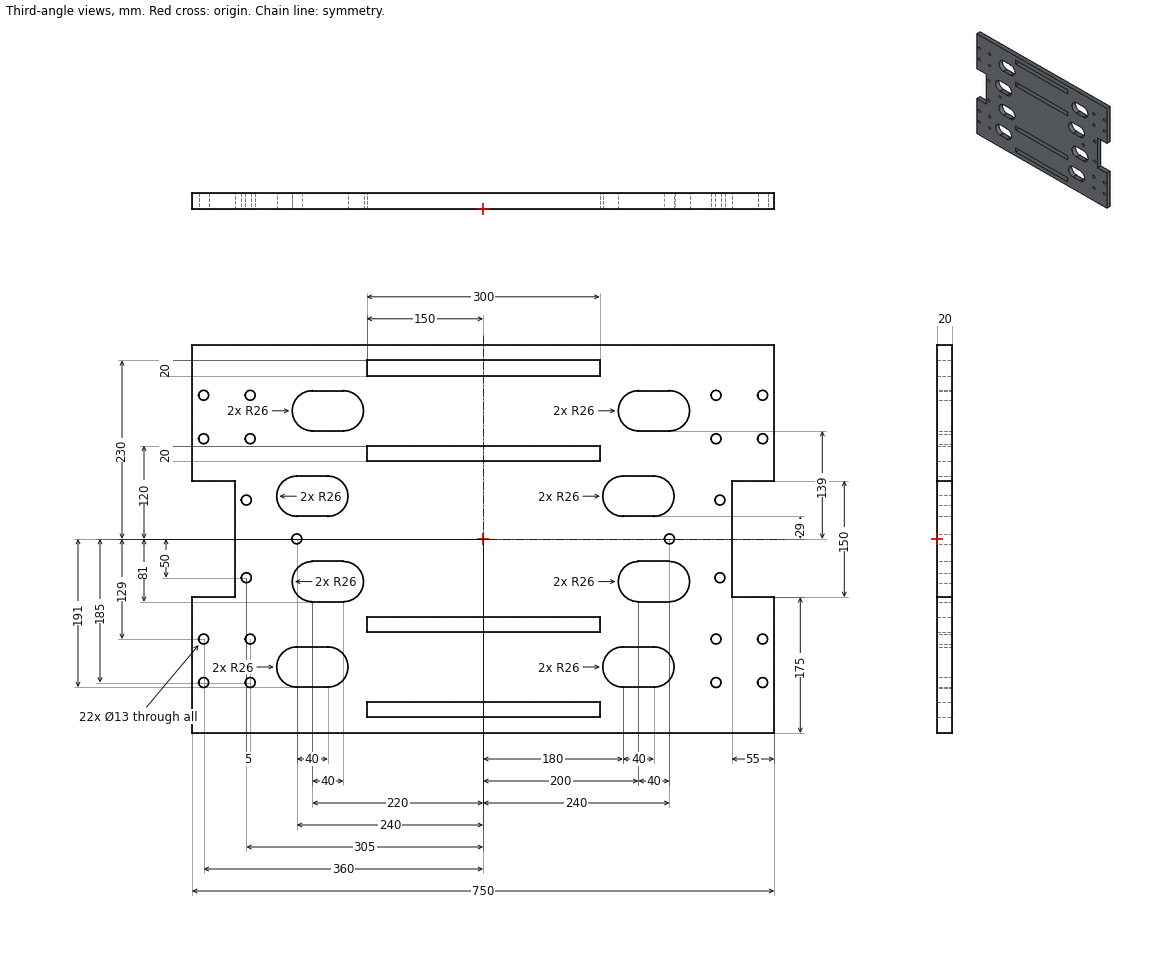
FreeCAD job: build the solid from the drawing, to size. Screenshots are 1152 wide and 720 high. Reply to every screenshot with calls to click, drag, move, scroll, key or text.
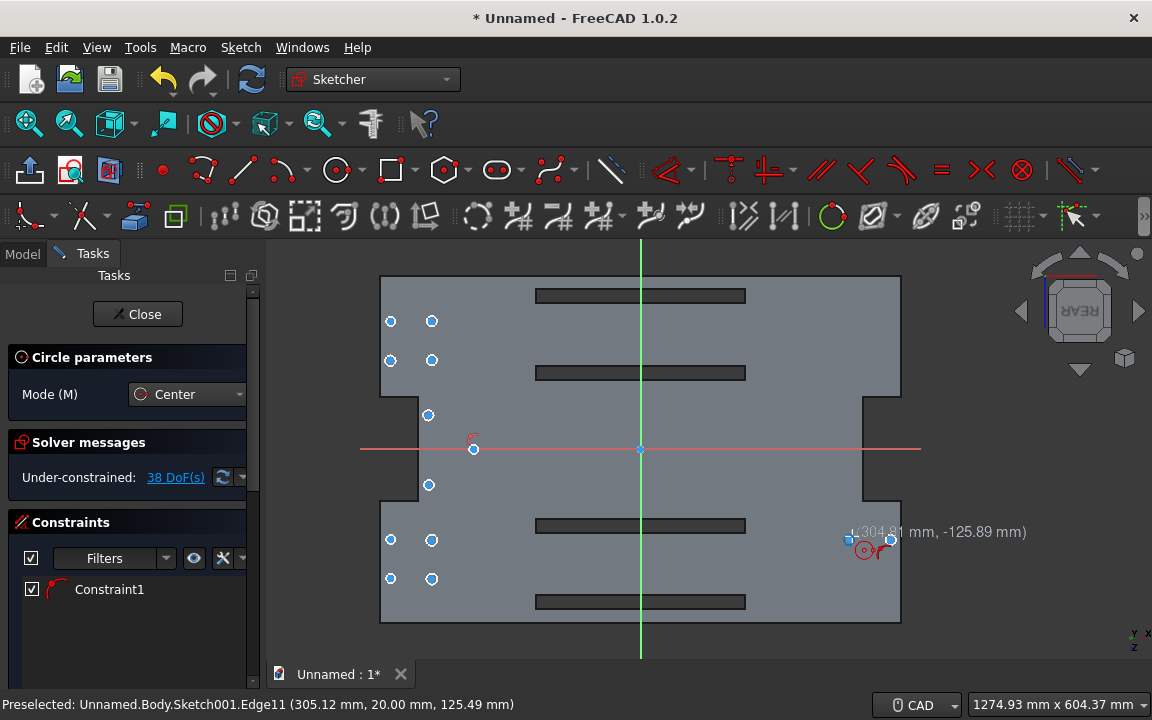
scroll(891, 578, up, 9)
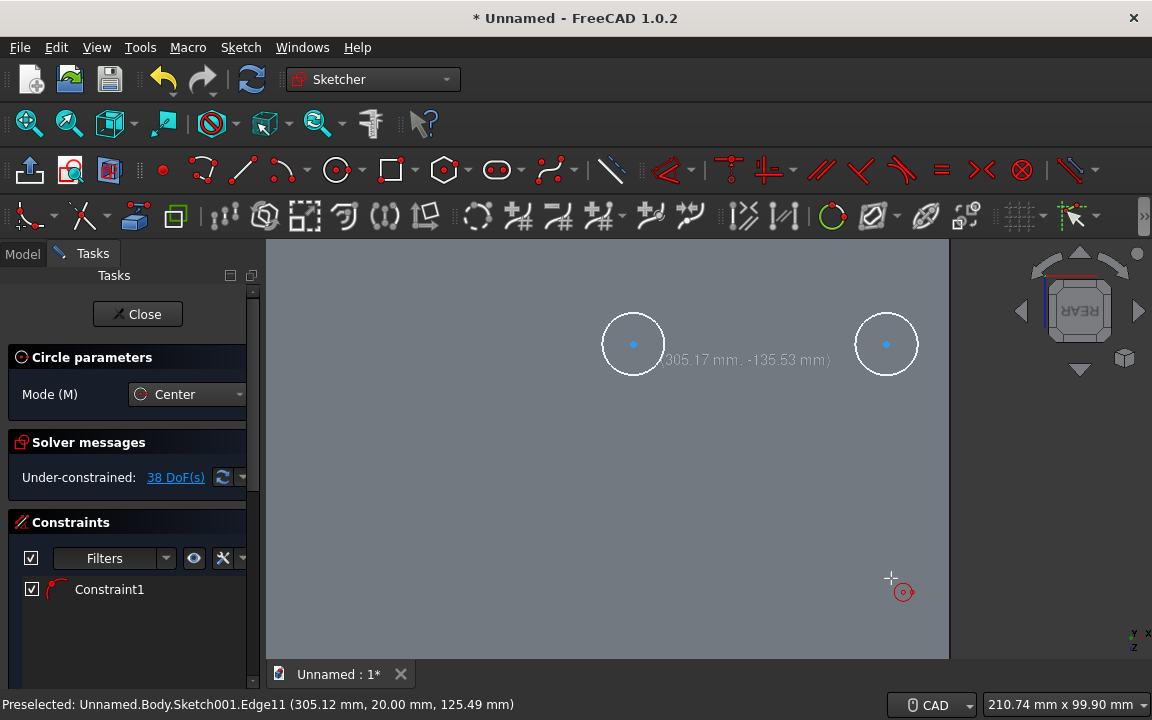
scroll(891, 578, down, 9)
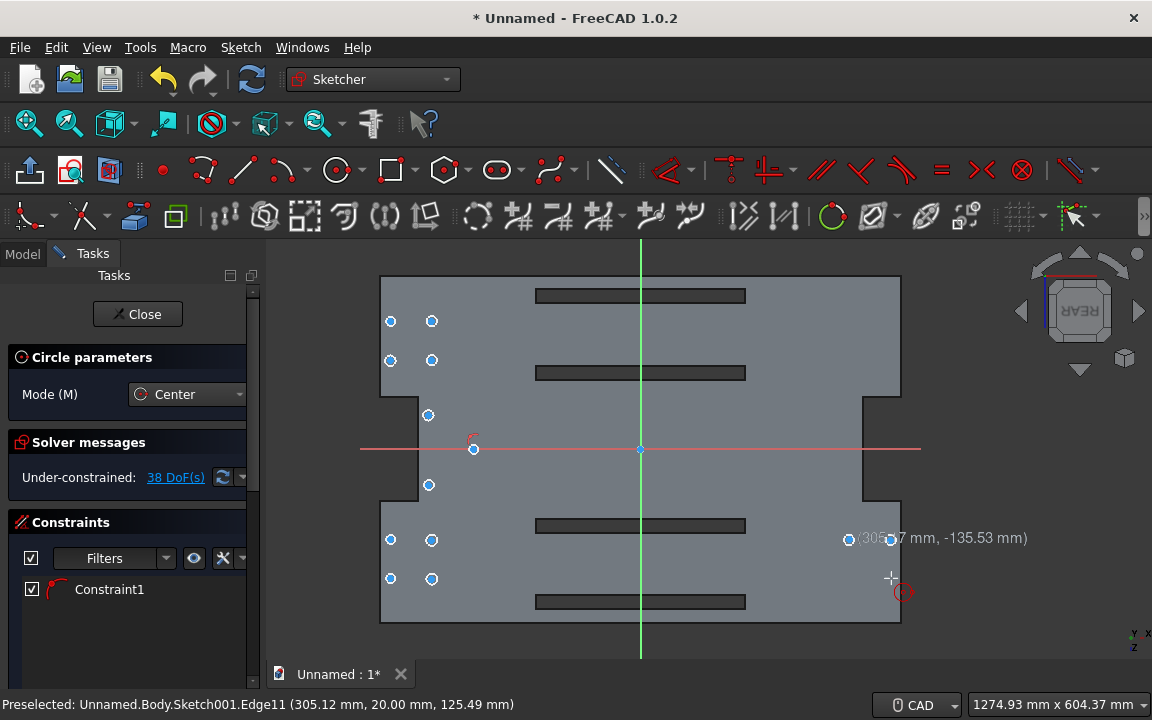
click(891, 578)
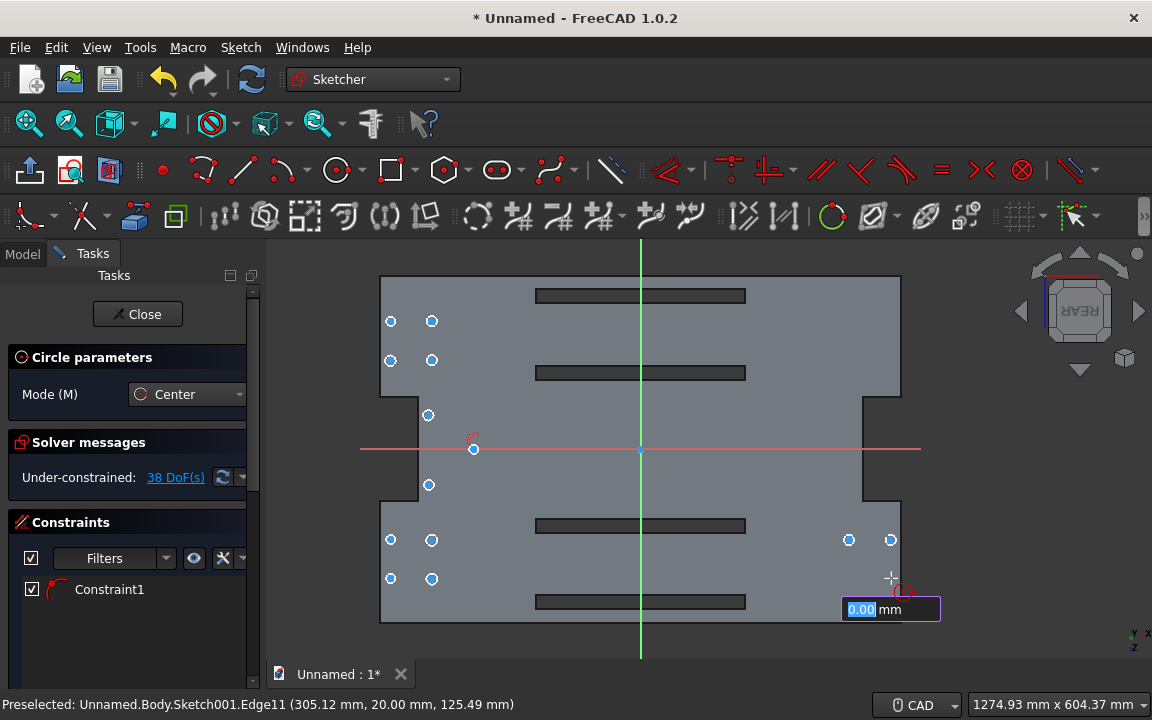
scroll(894, 575, up, 7)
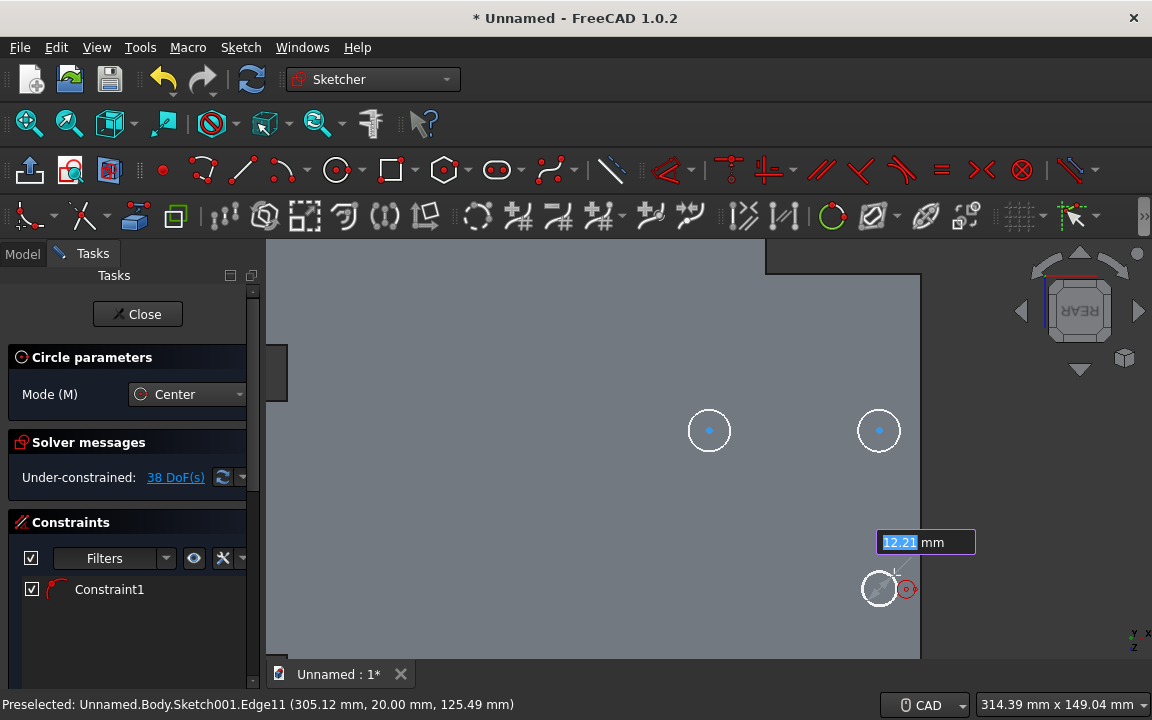
click(892, 571)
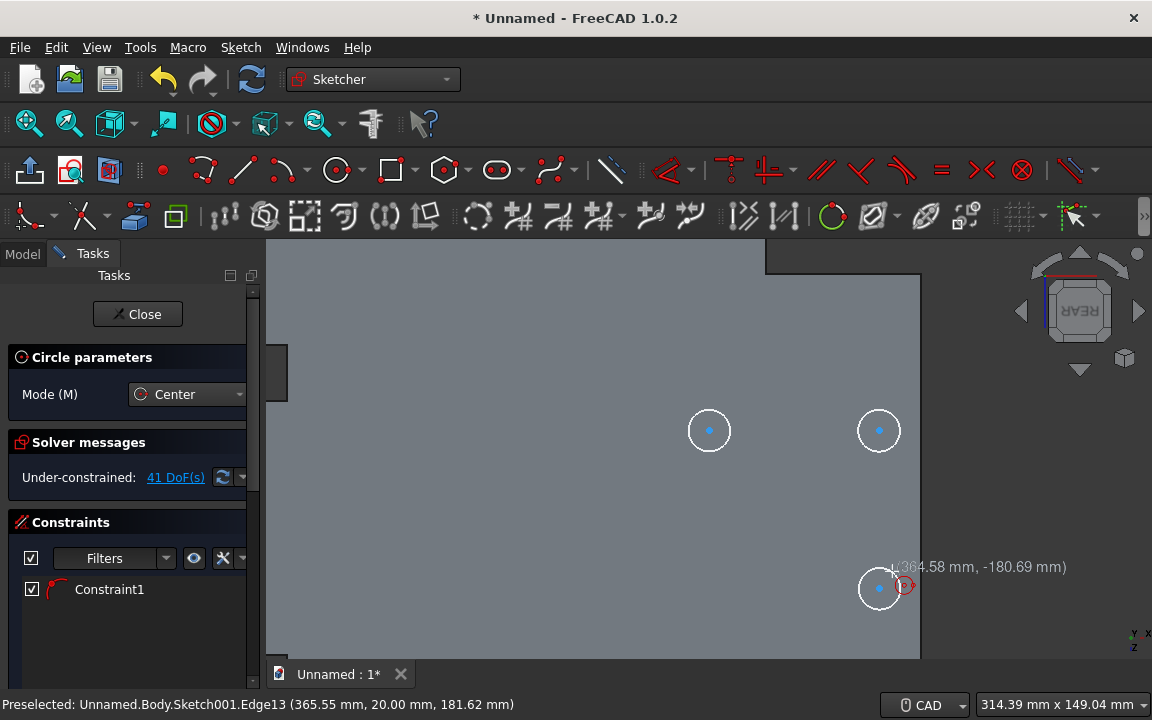
scroll(894, 575, down, 7)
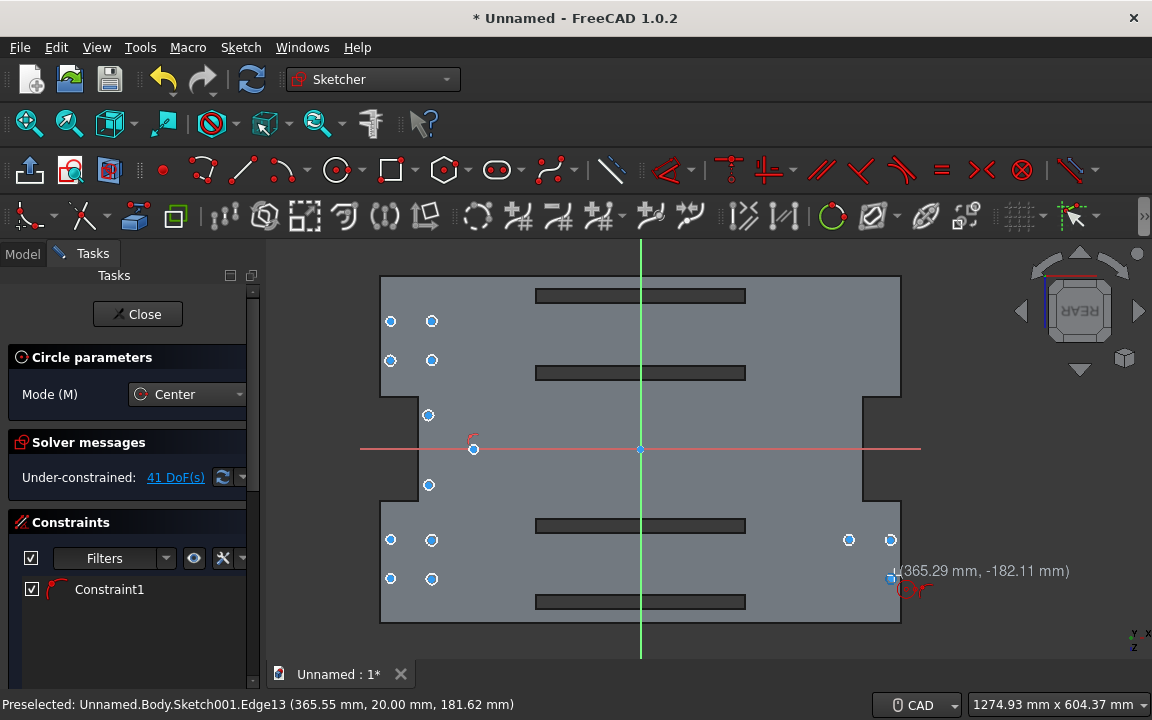
scroll(891, 360, up, 9)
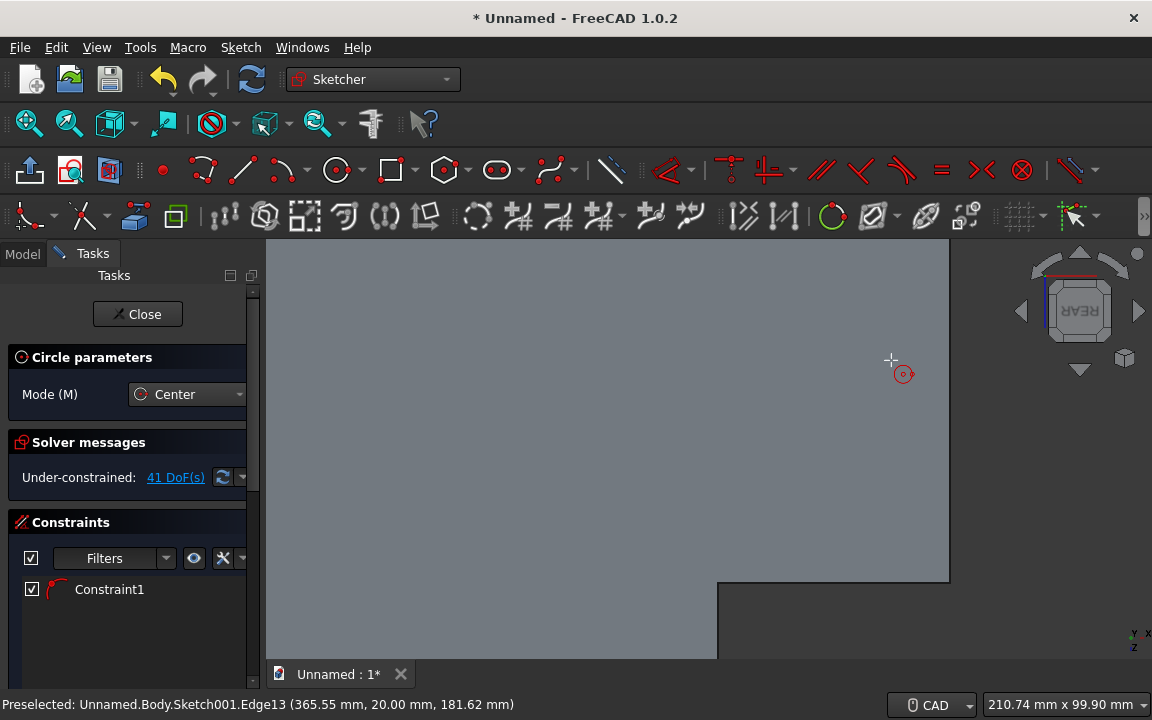
scroll(891, 360, down, 9)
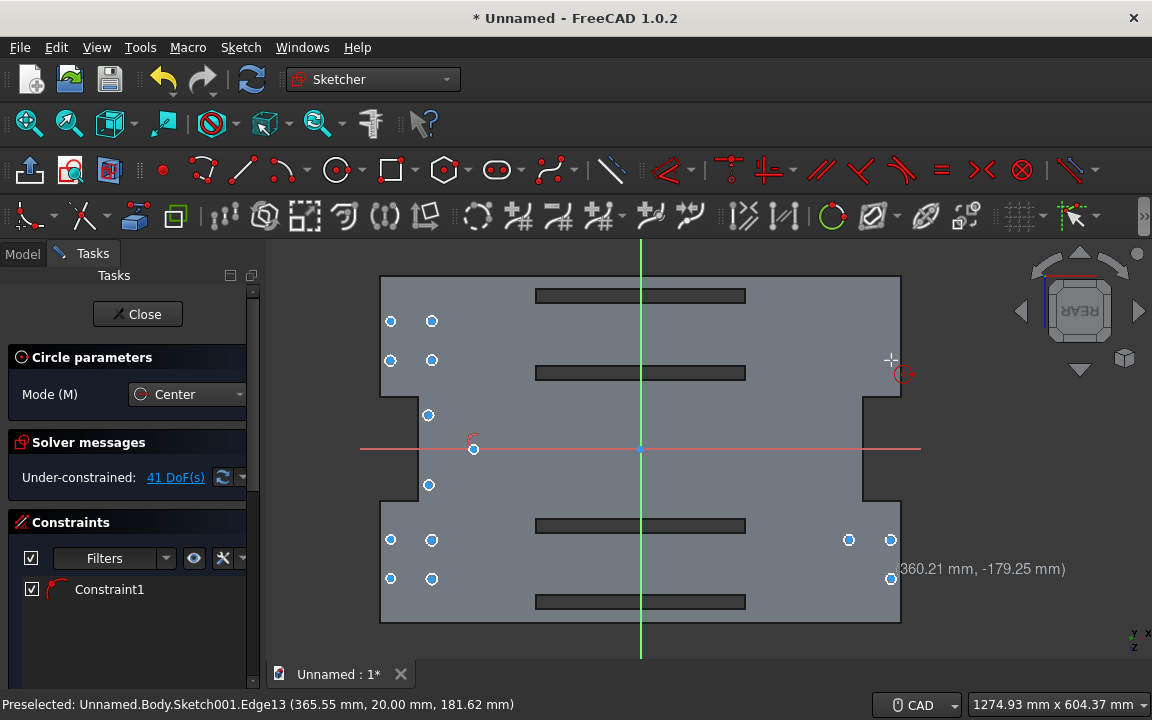
click(891, 360)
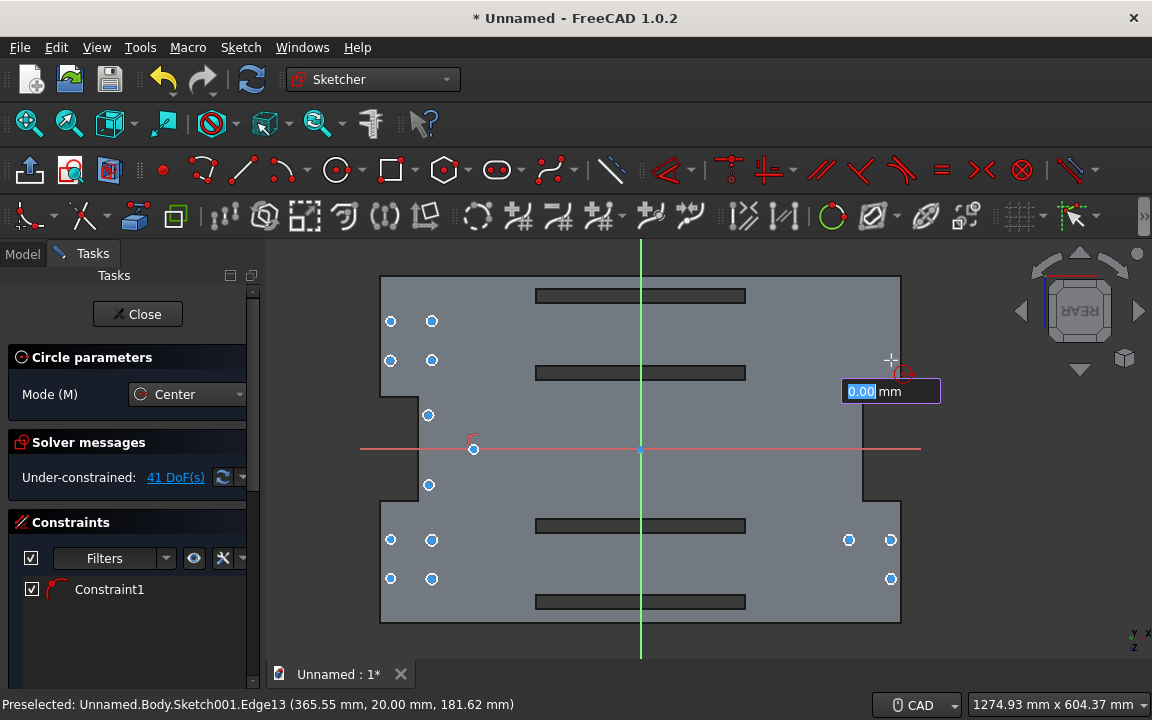
scroll(894, 356, up, 7)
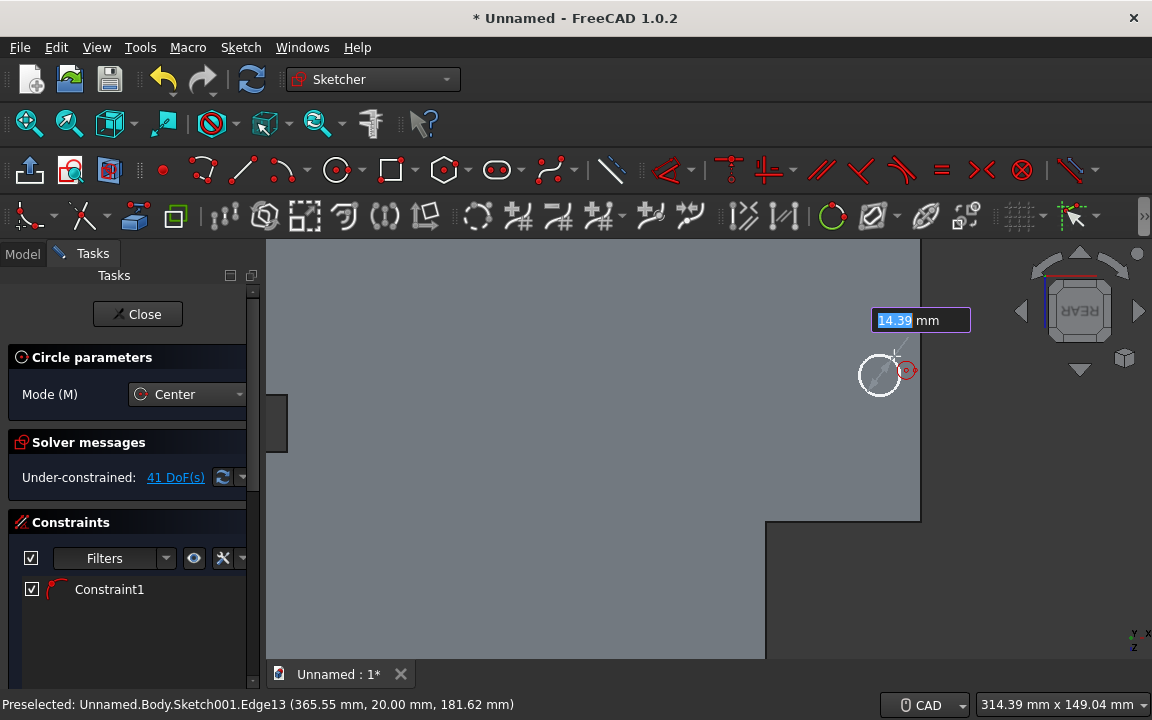
click(892, 357)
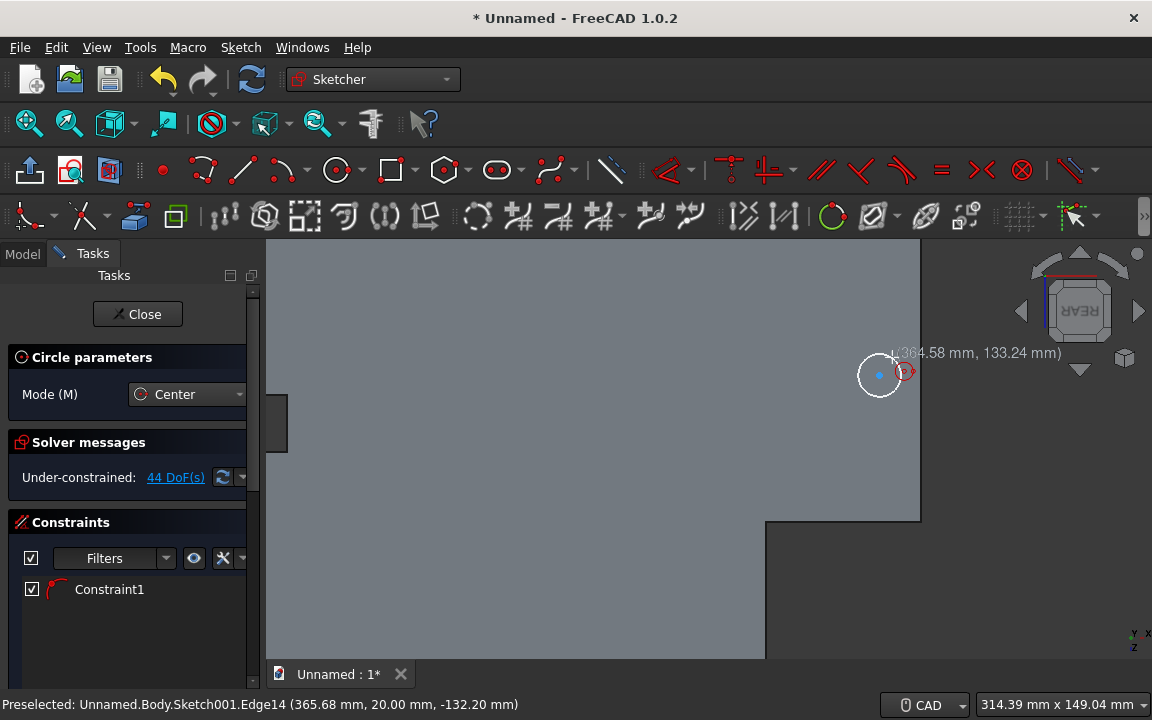
scroll(894, 356, down, 7)